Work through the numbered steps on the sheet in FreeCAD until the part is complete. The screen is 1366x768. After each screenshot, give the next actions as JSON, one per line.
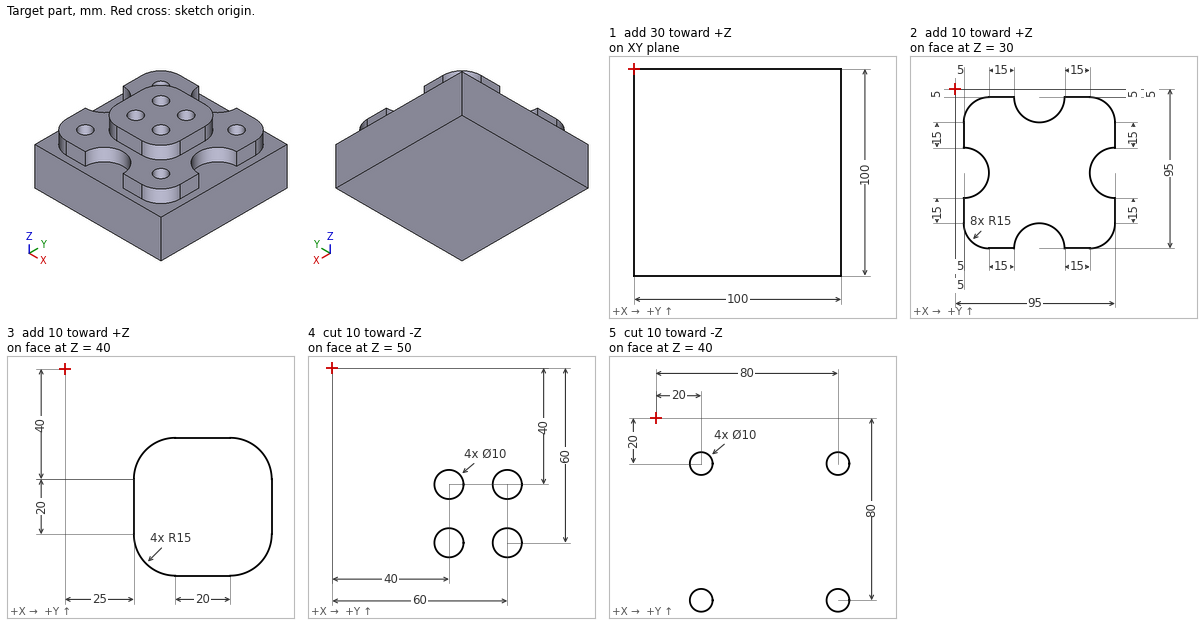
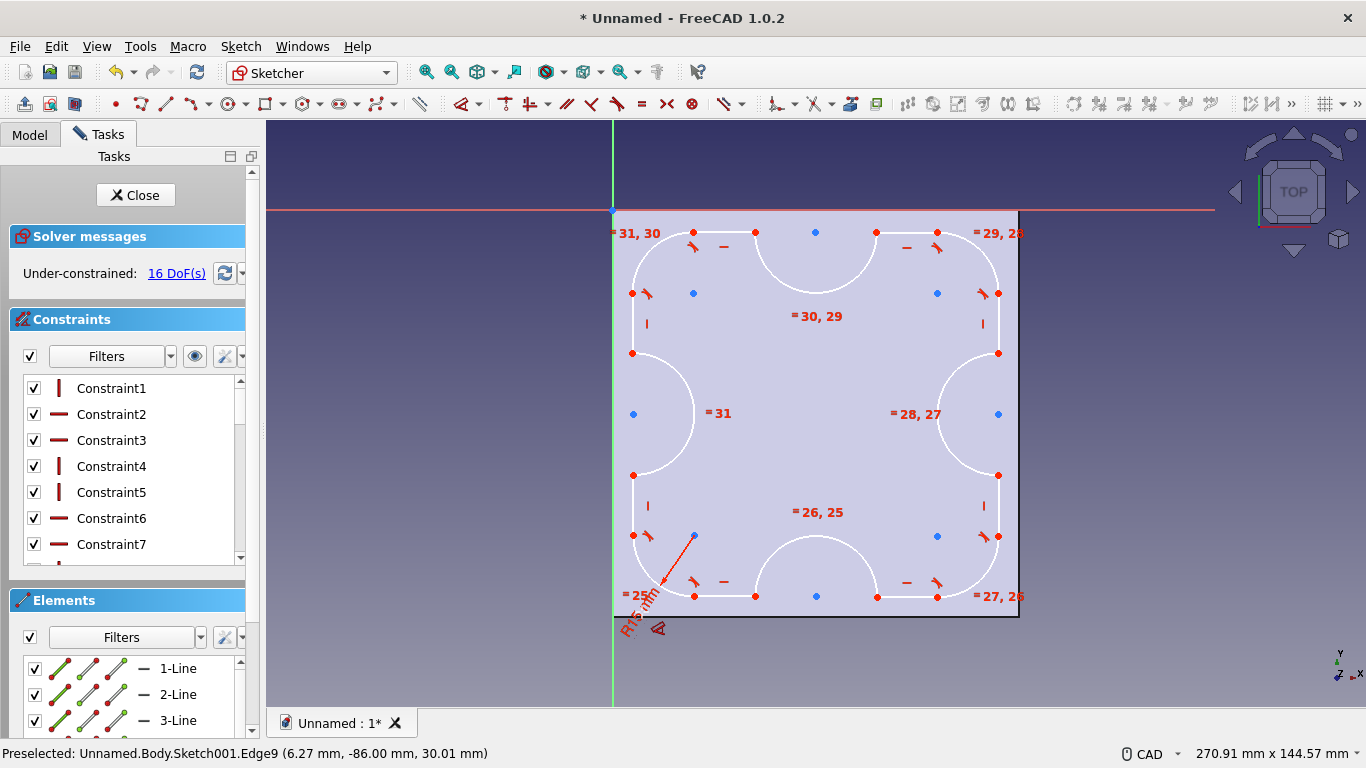
{"action": "left_click", "coordinate": [633, 493]}
{"action": "left_click", "coordinate": [599, 505]}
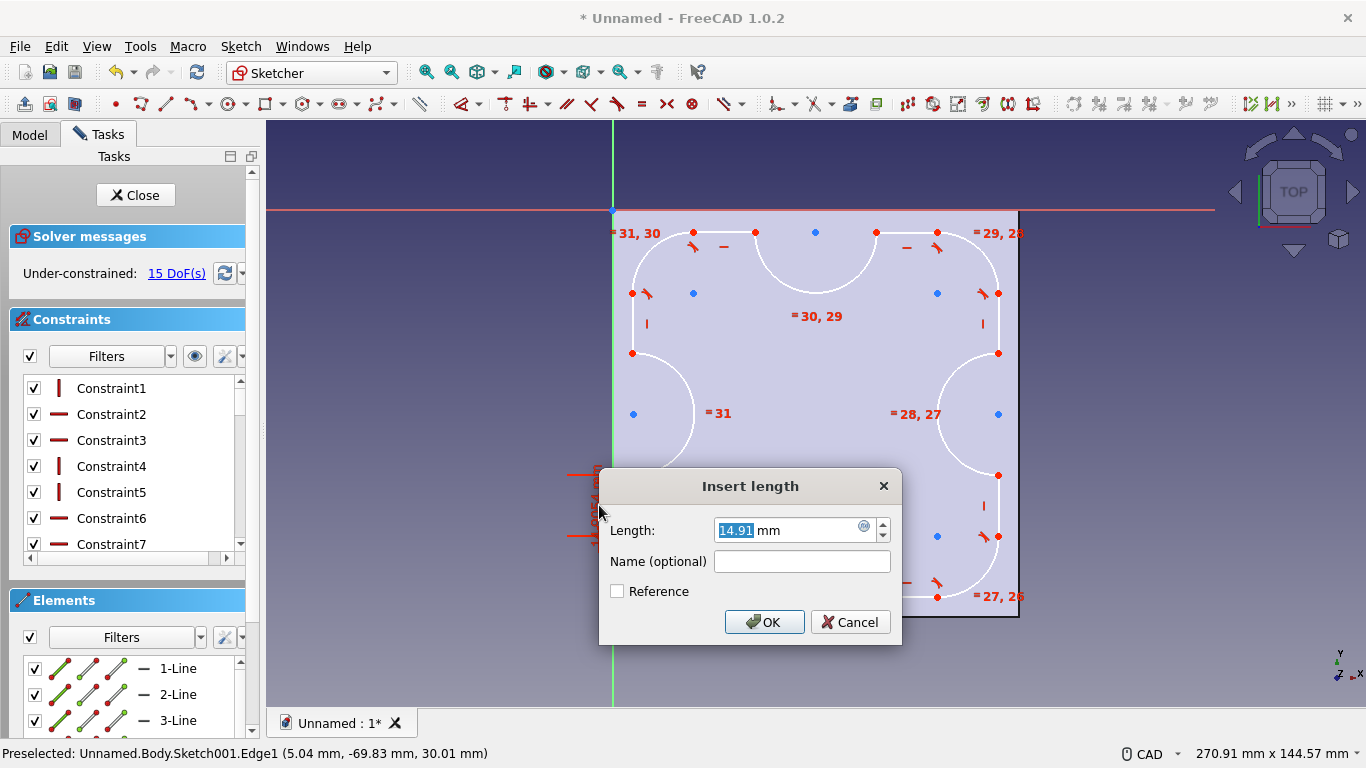
{"action": "type", "text": "15"}
{"action": "key", "text": "Return"}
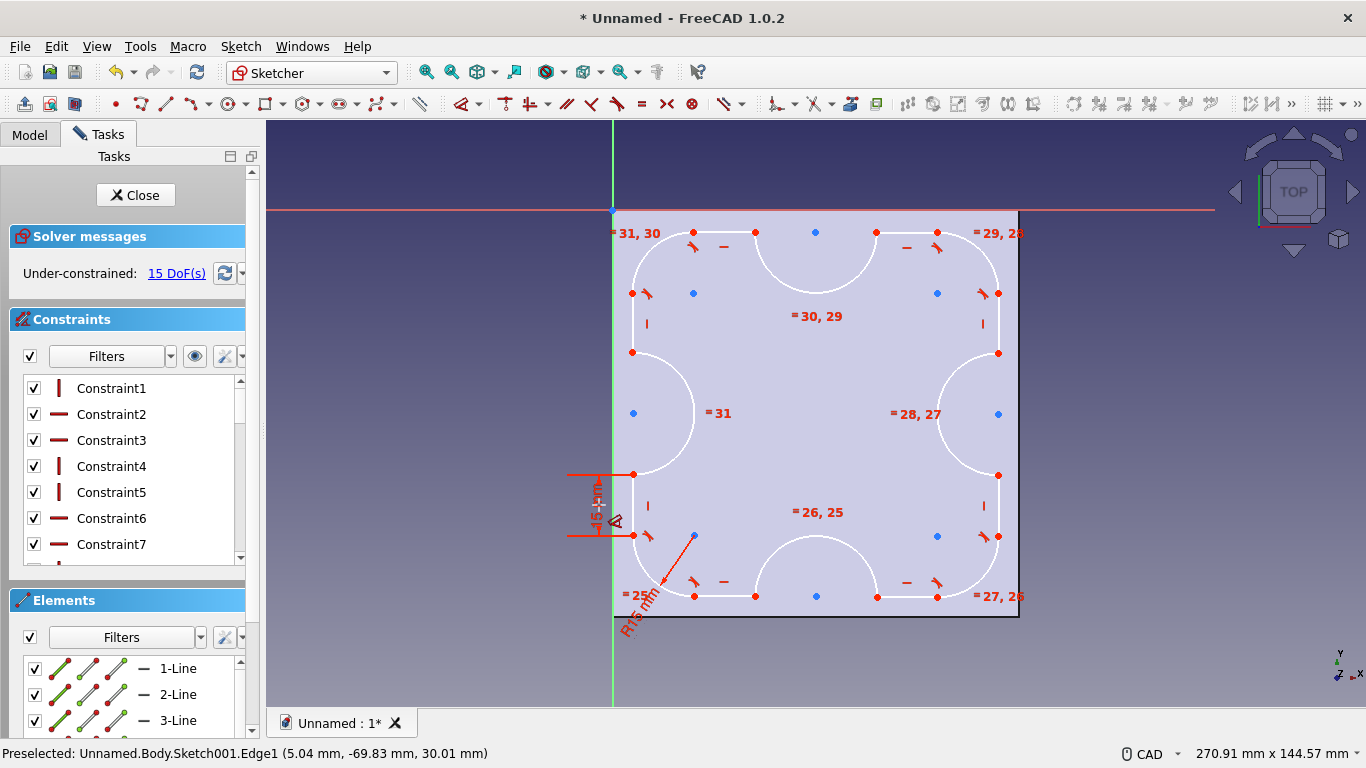
{"action": "left_click", "coordinate": [713, 596]}
{"action": "left_click", "coordinate": [725, 630]}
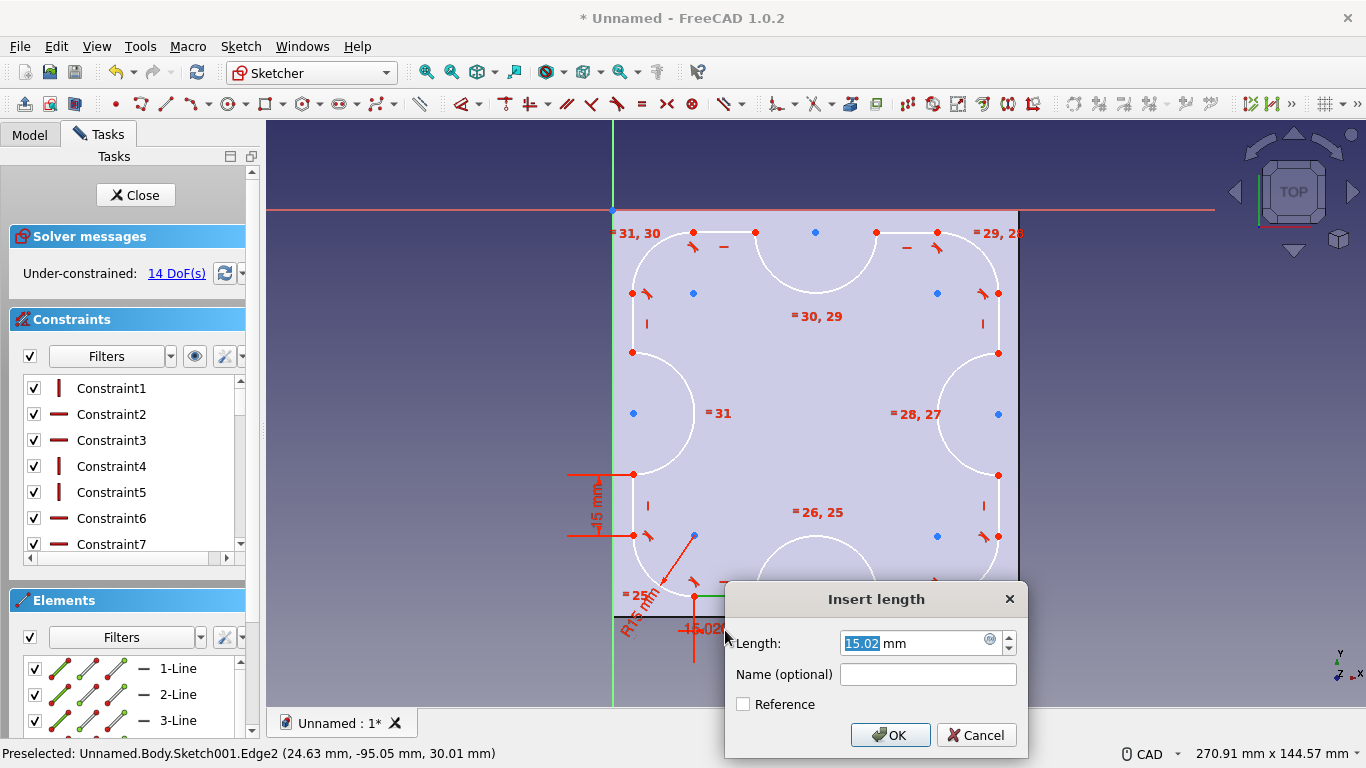
{"action": "type", "text": "15"}
{"action": "key", "text": "Return"}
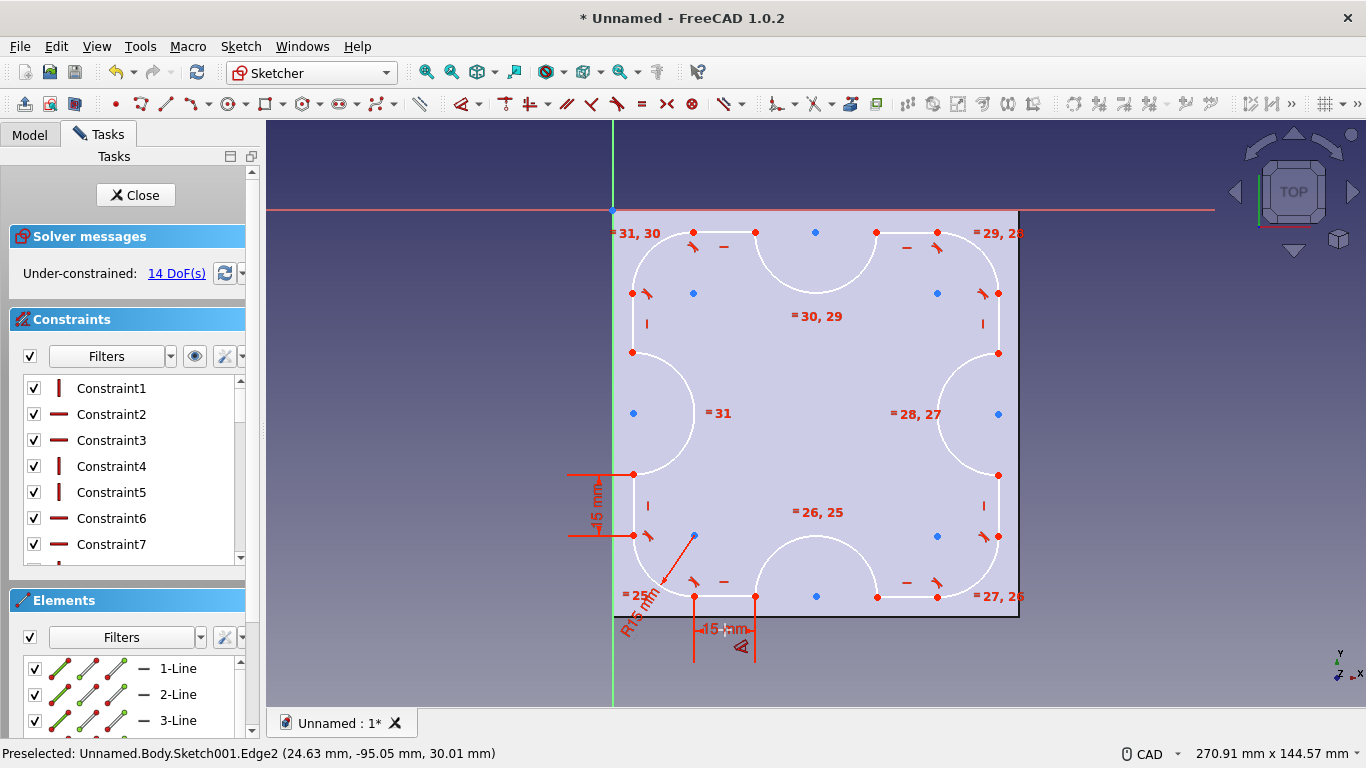
{"action": "left_click", "coordinate": [895, 597]}
{"action": "left_click", "coordinate": [907, 631]}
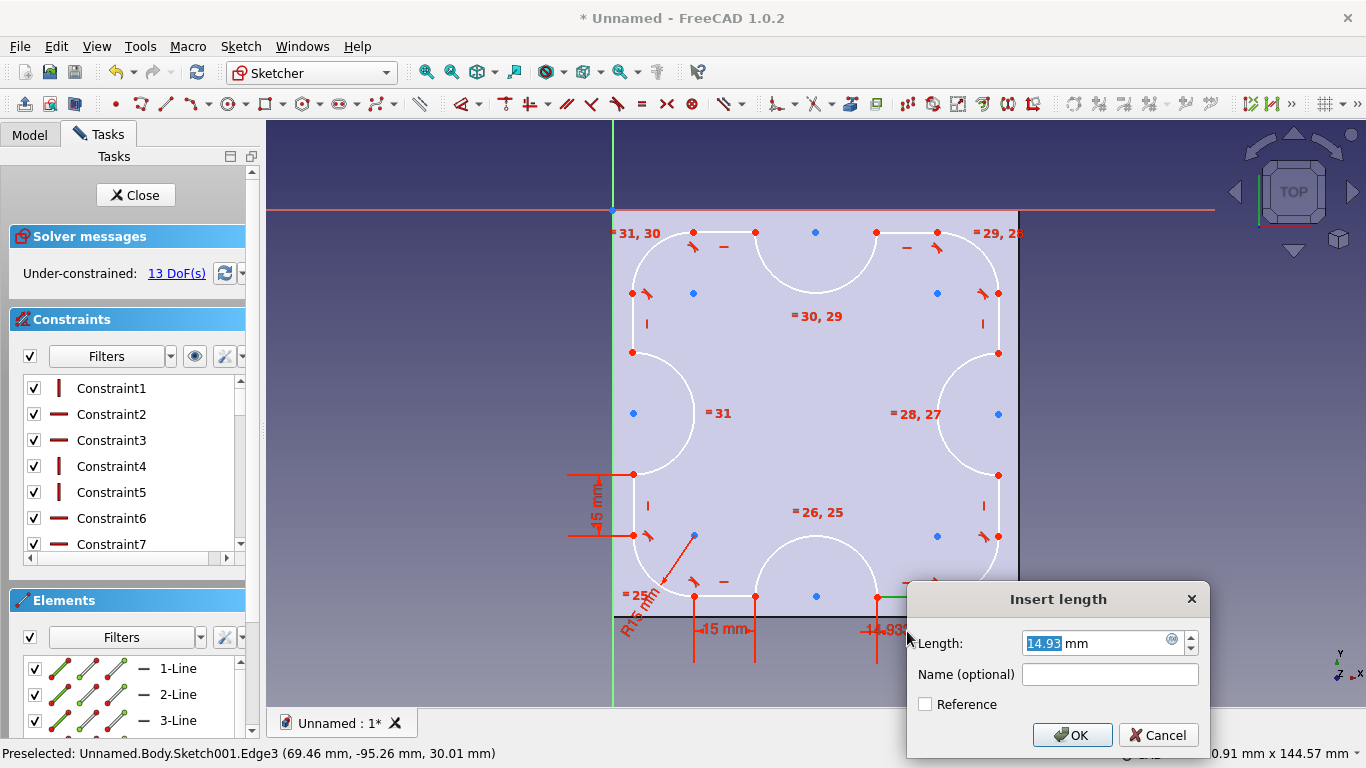
{"action": "type", "text": "15"}
{"action": "key", "text": "Return"}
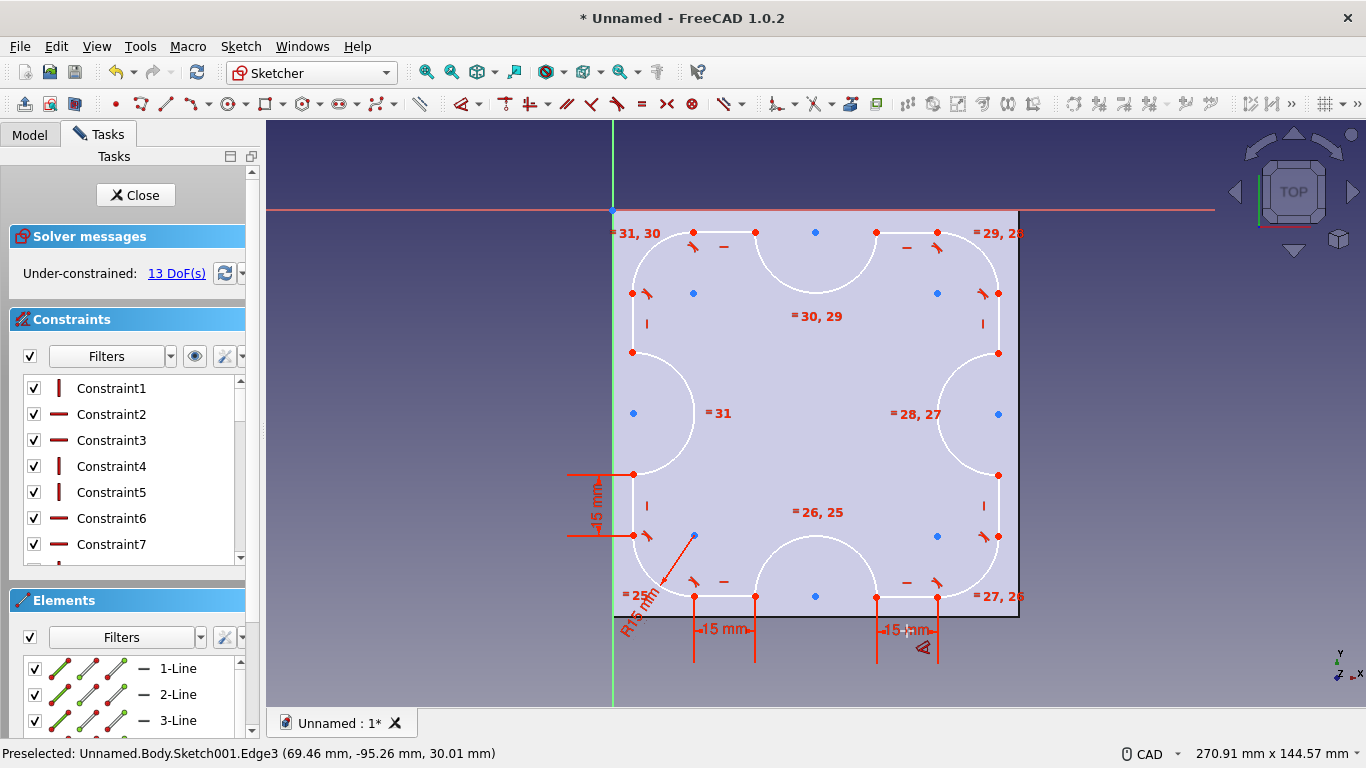
{"action": "left_click", "coordinate": [999, 518]}
{"action": "left_click", "coordinate": [1033, 506]}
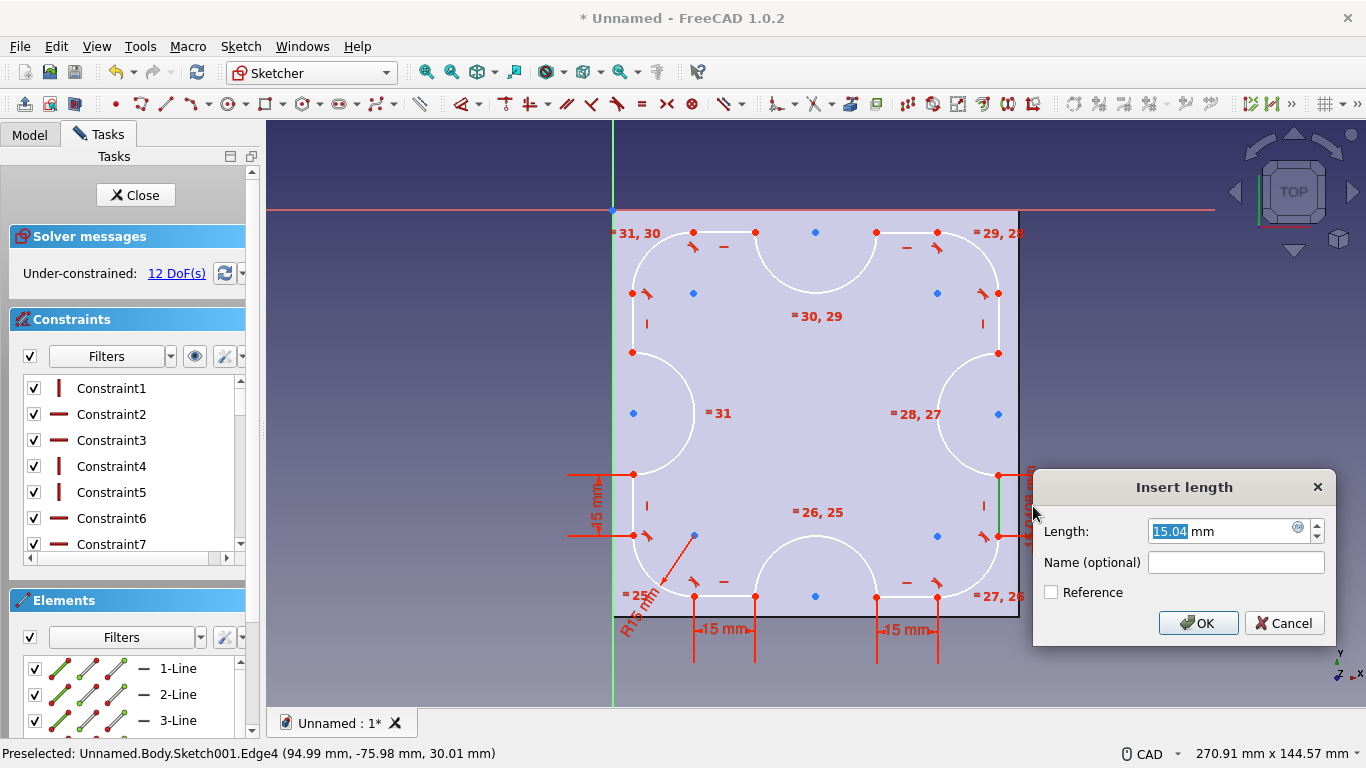
{"action": "type", "text": "15"}
{"action": "key", "text": "Return"}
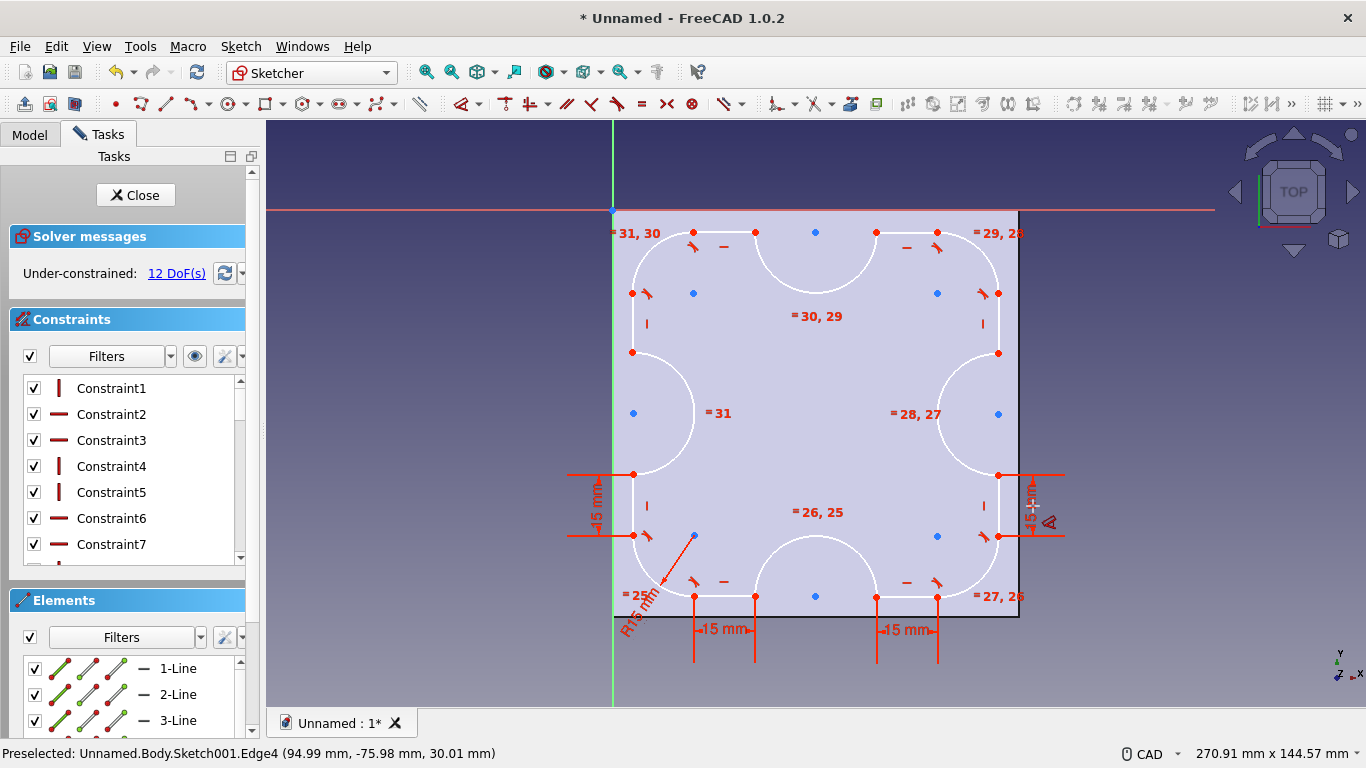
{"action": "left_click", "coordinate": [999, 336]}
{"action": "left_click", "coordinate": [1033, 324]}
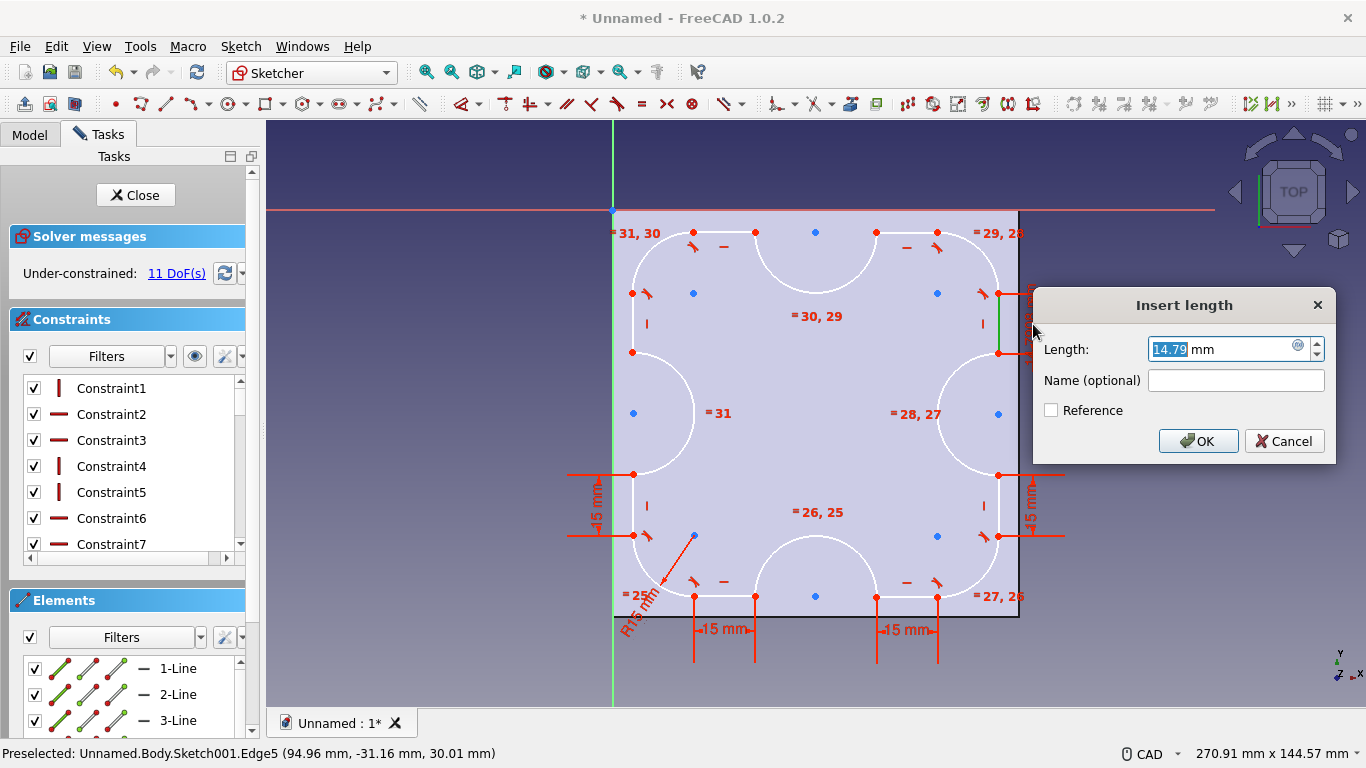
{"action": "type", "text": "15"}
{"action": "key", "text": "Return"}